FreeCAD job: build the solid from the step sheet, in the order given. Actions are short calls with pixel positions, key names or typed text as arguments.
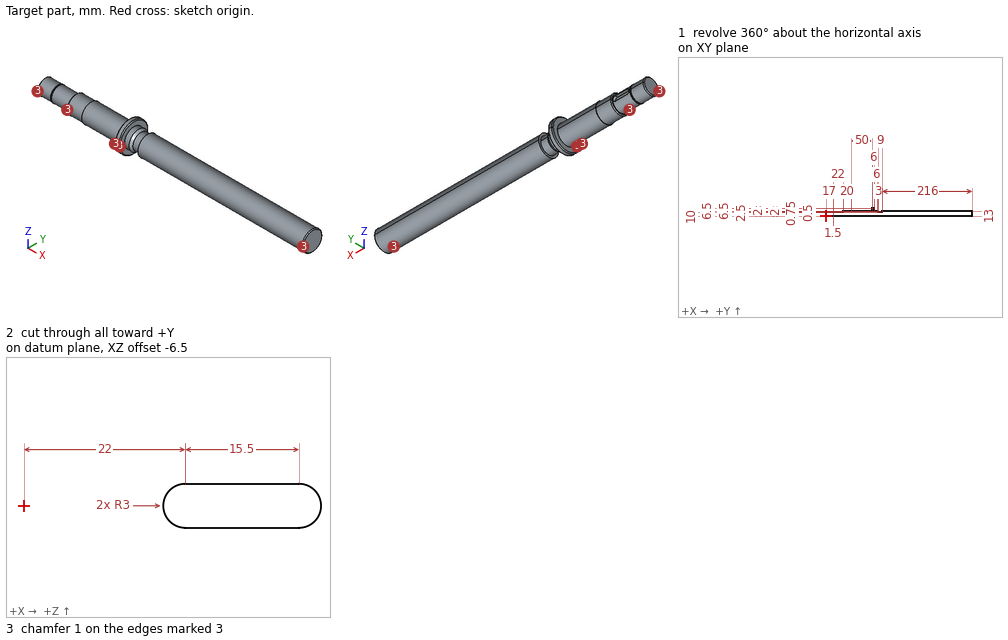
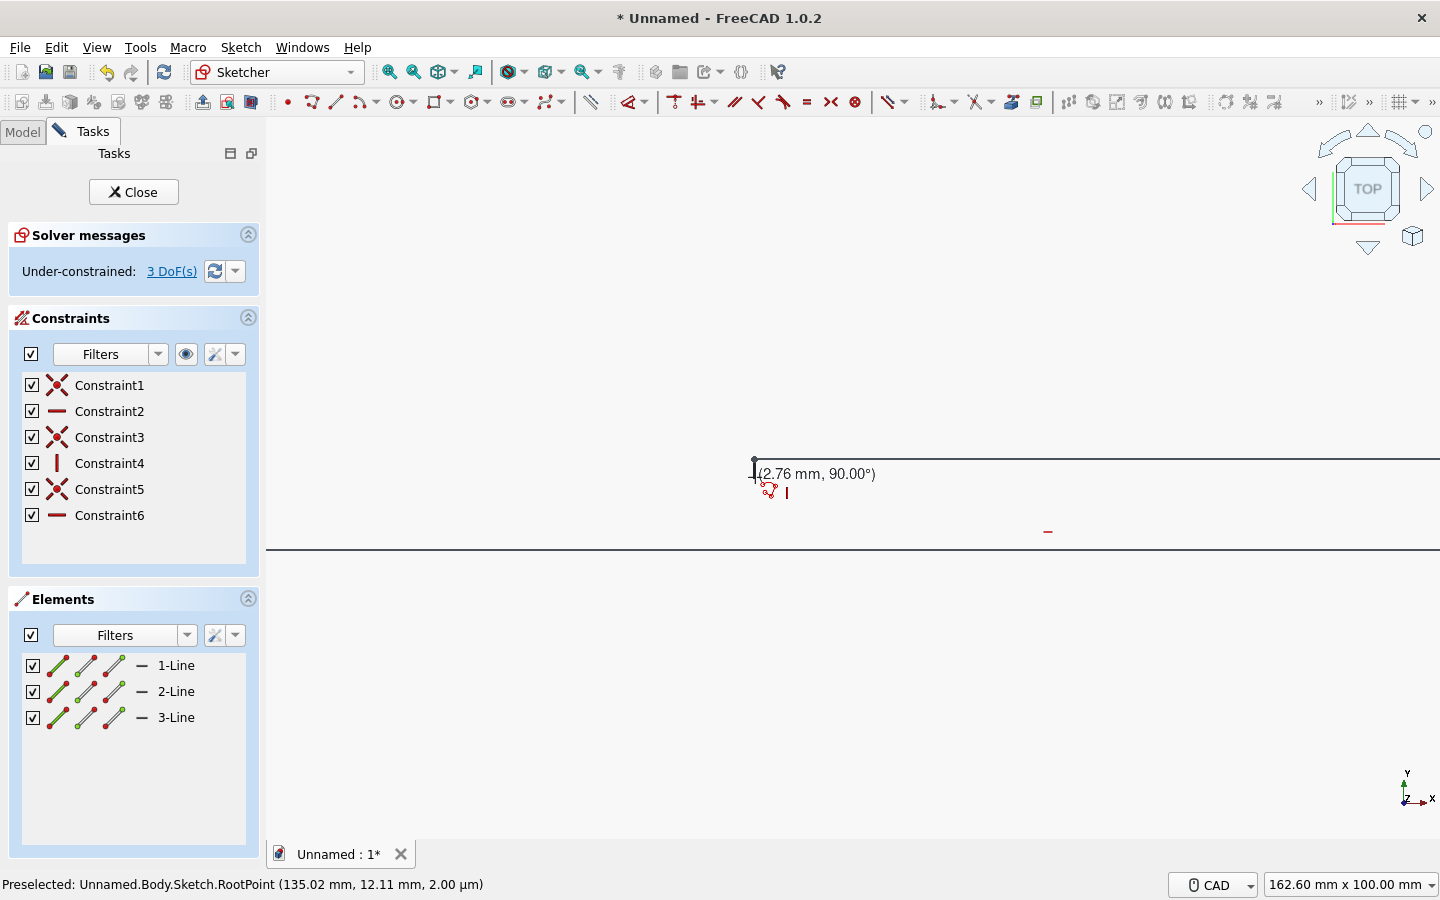
click(754, 474)
click(689, 474)
click(667, 460)
click(624, 460)
click(624, 413)
click(580, 413)
click(580, 460)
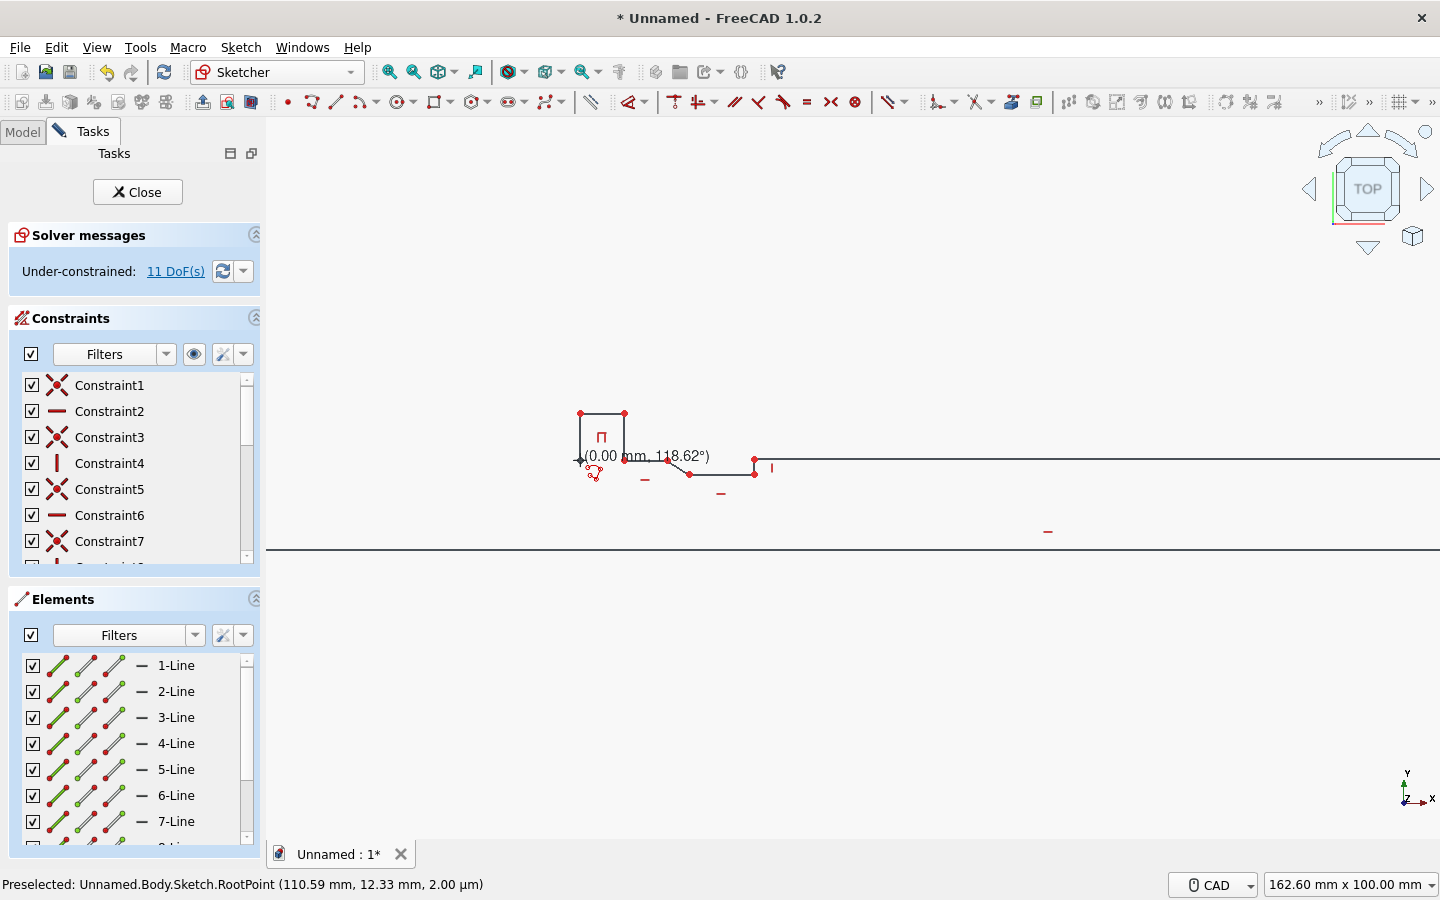
scroll(671, 477, down, 6)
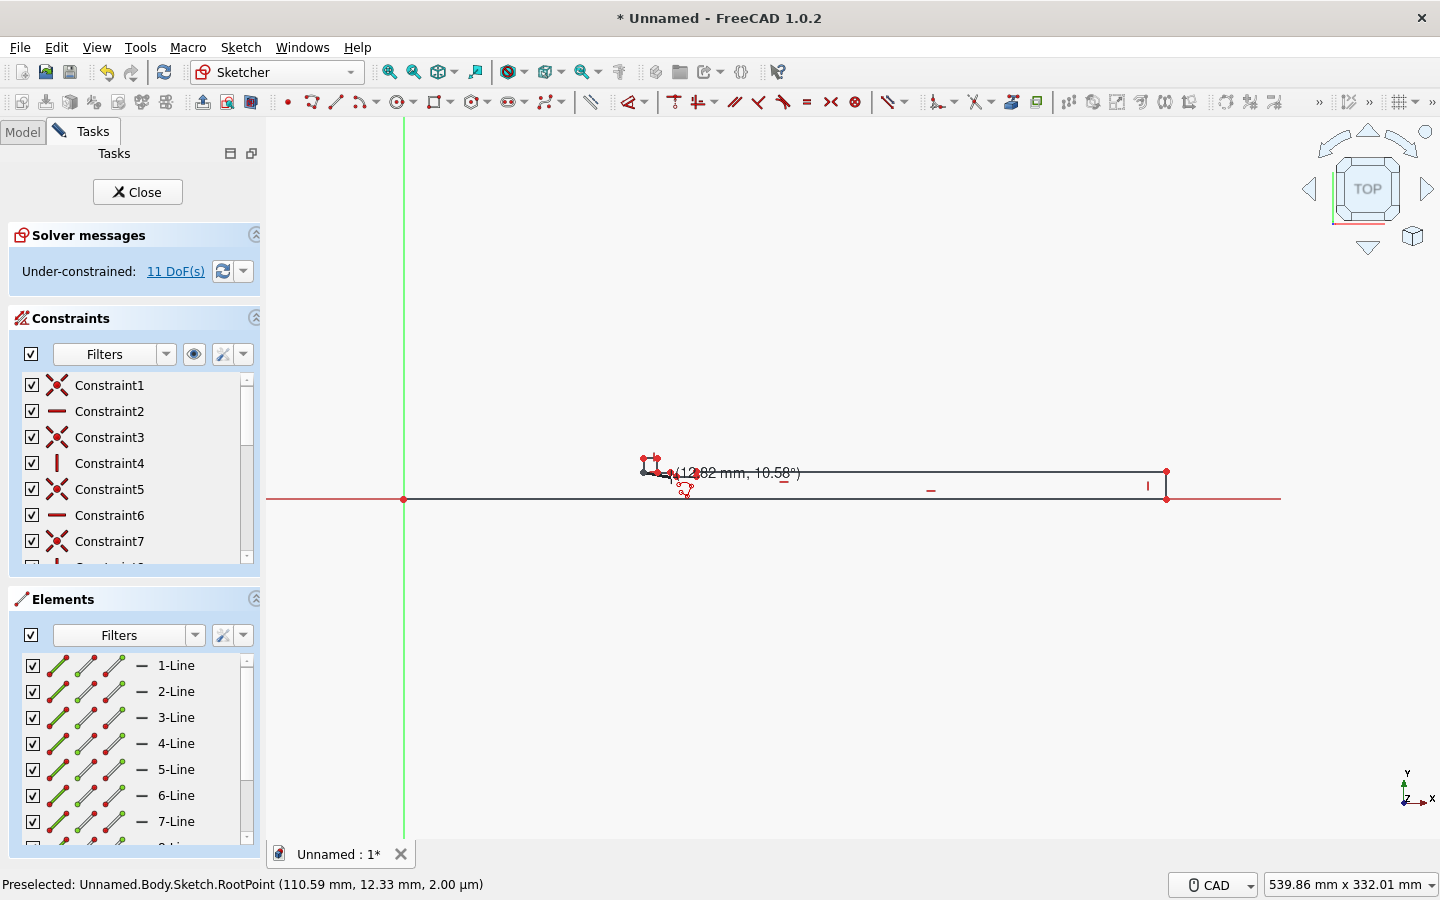
click(535, 472)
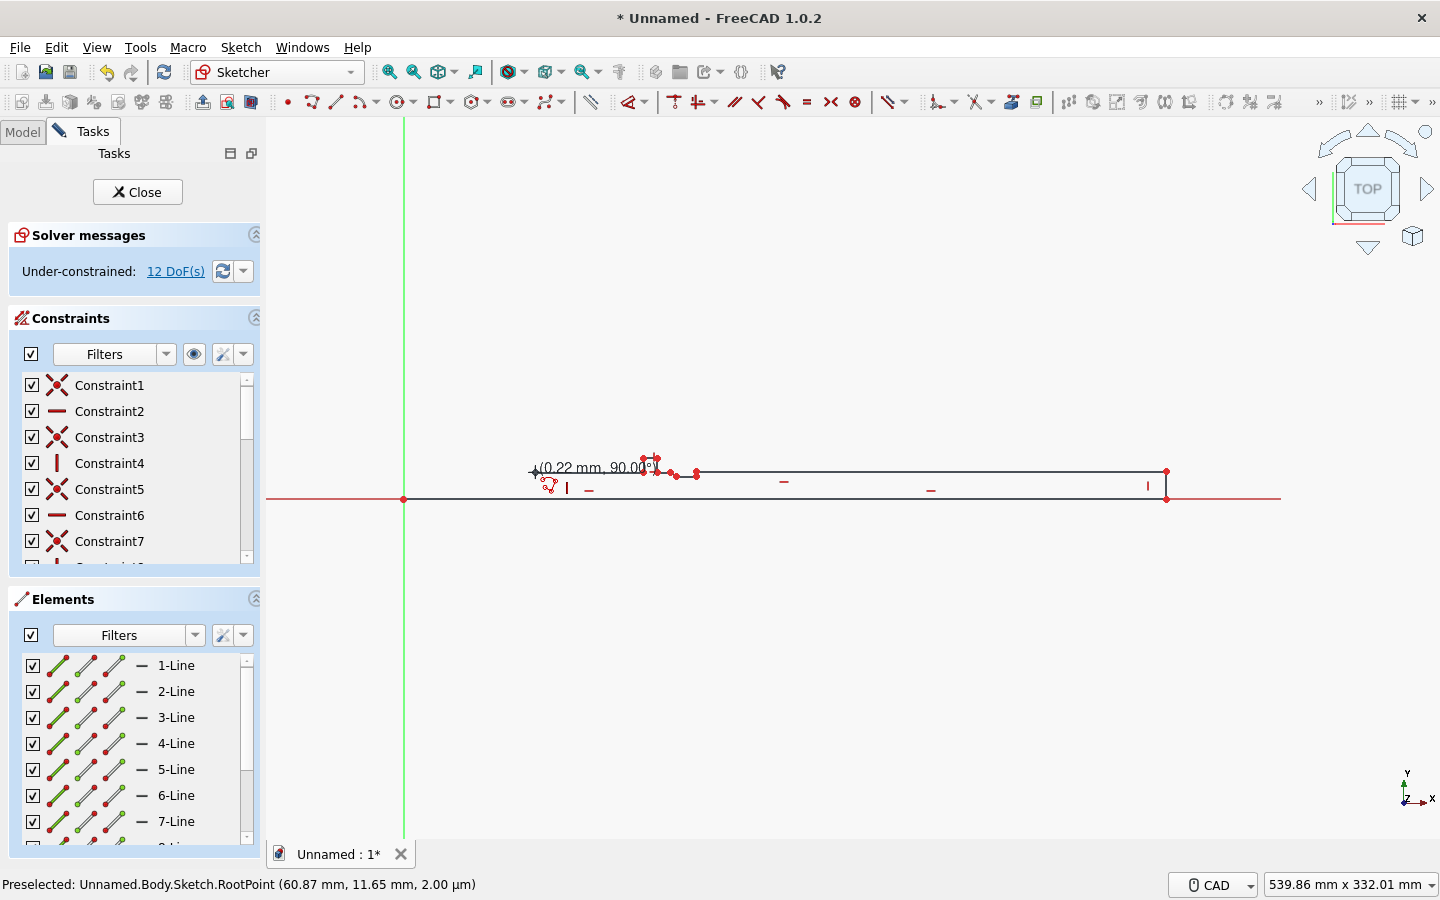
scroll(535, 473, up, 14)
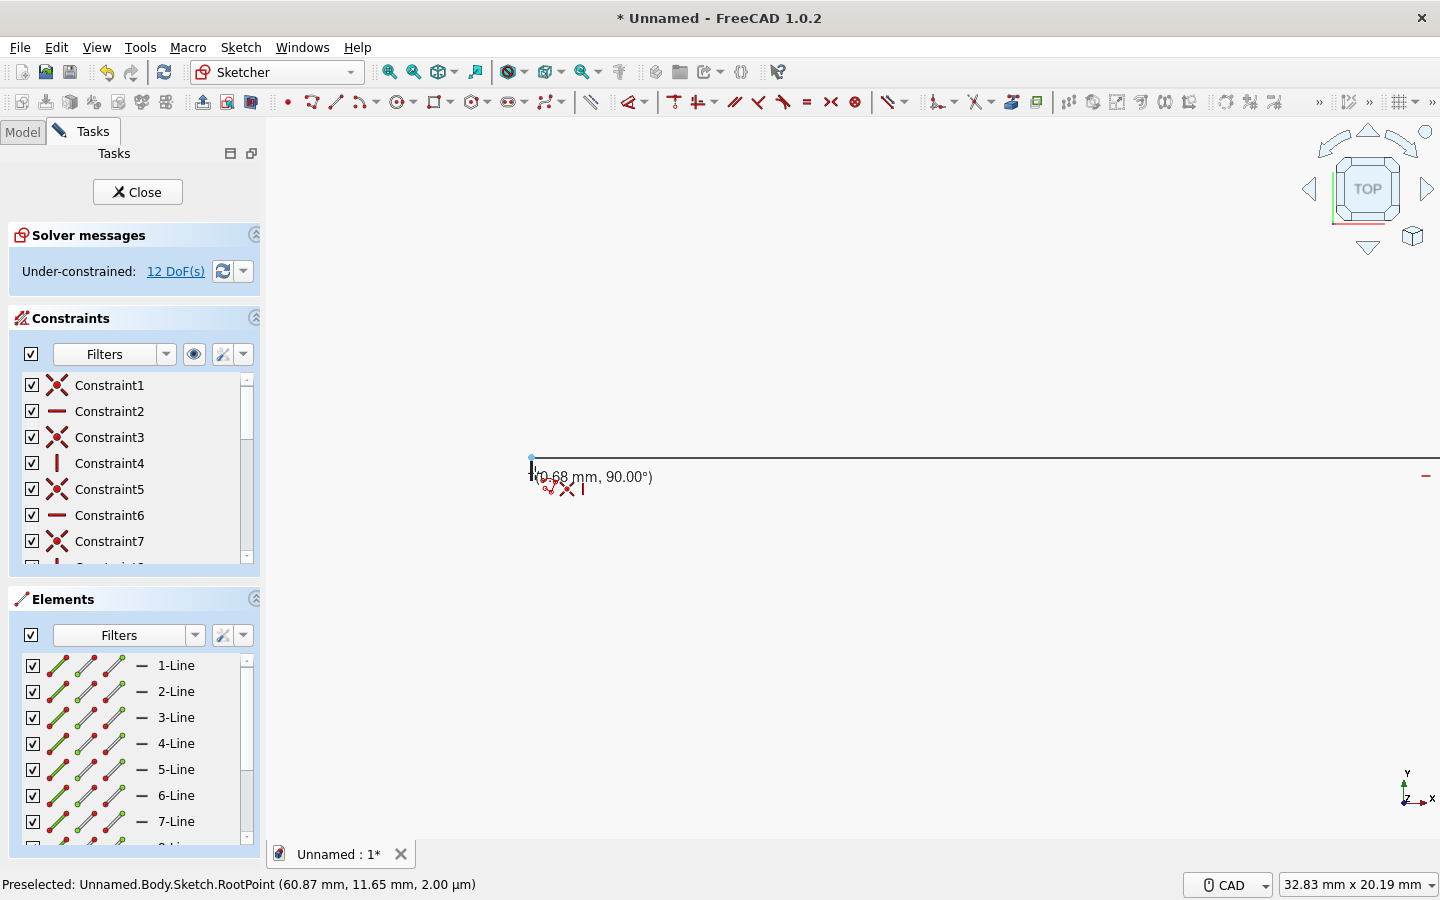
click(531, 469)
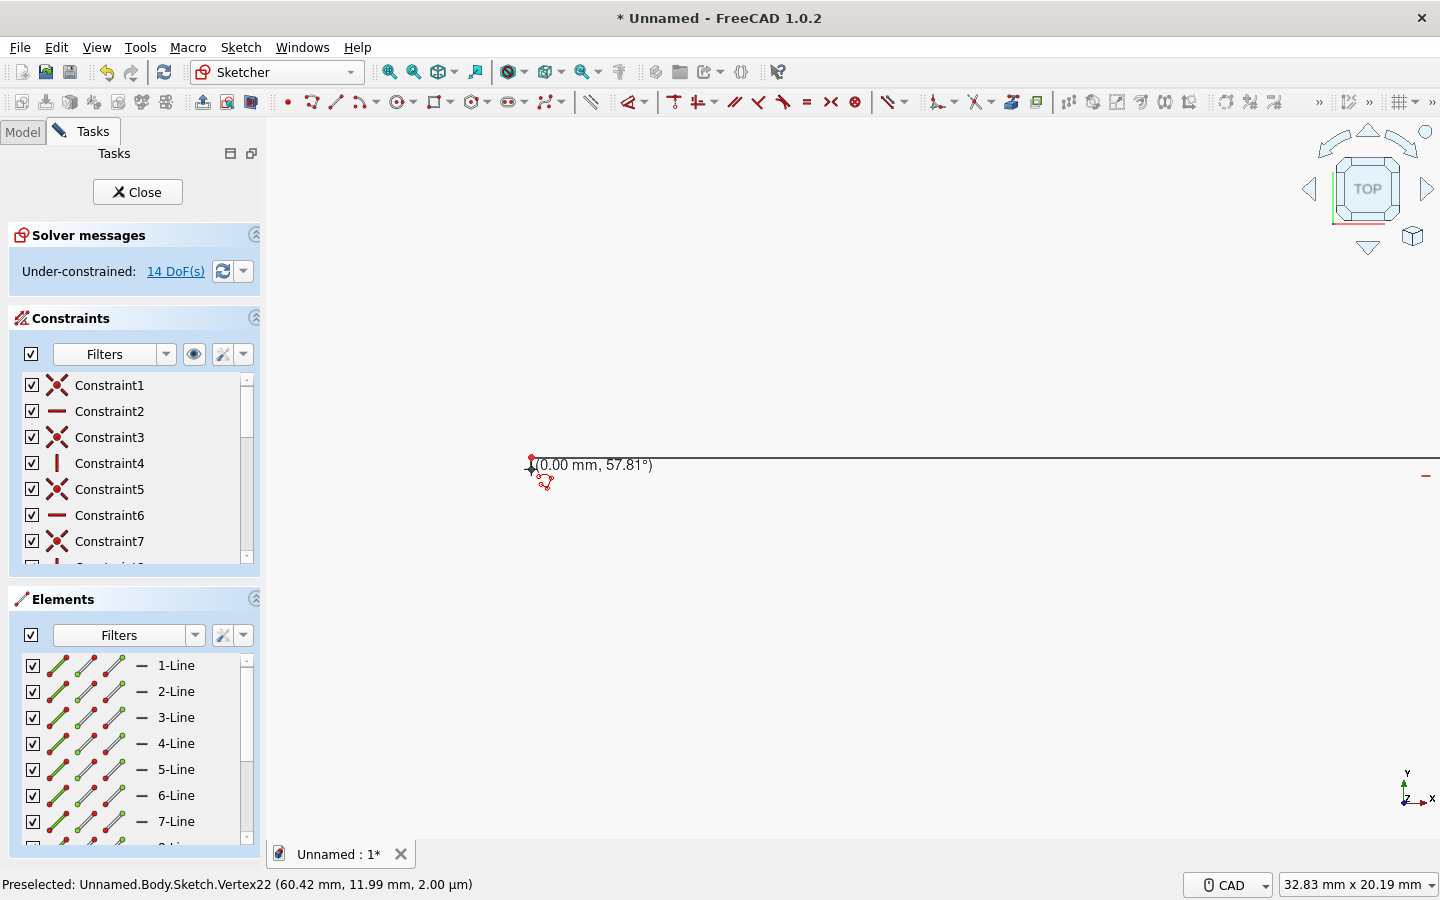
scroll(535, 473, down, 14)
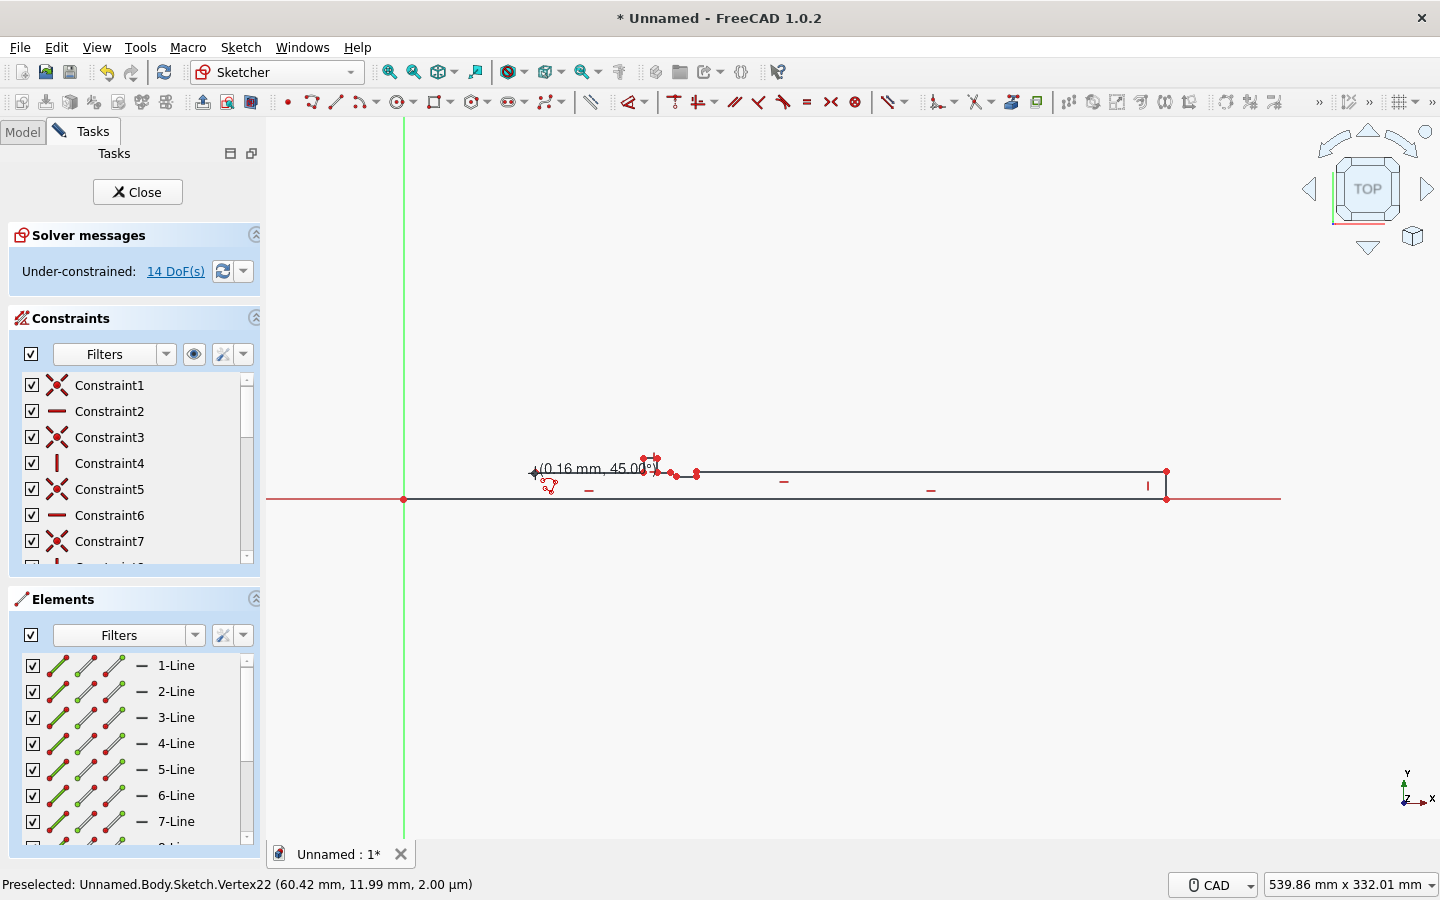
click(492, 473)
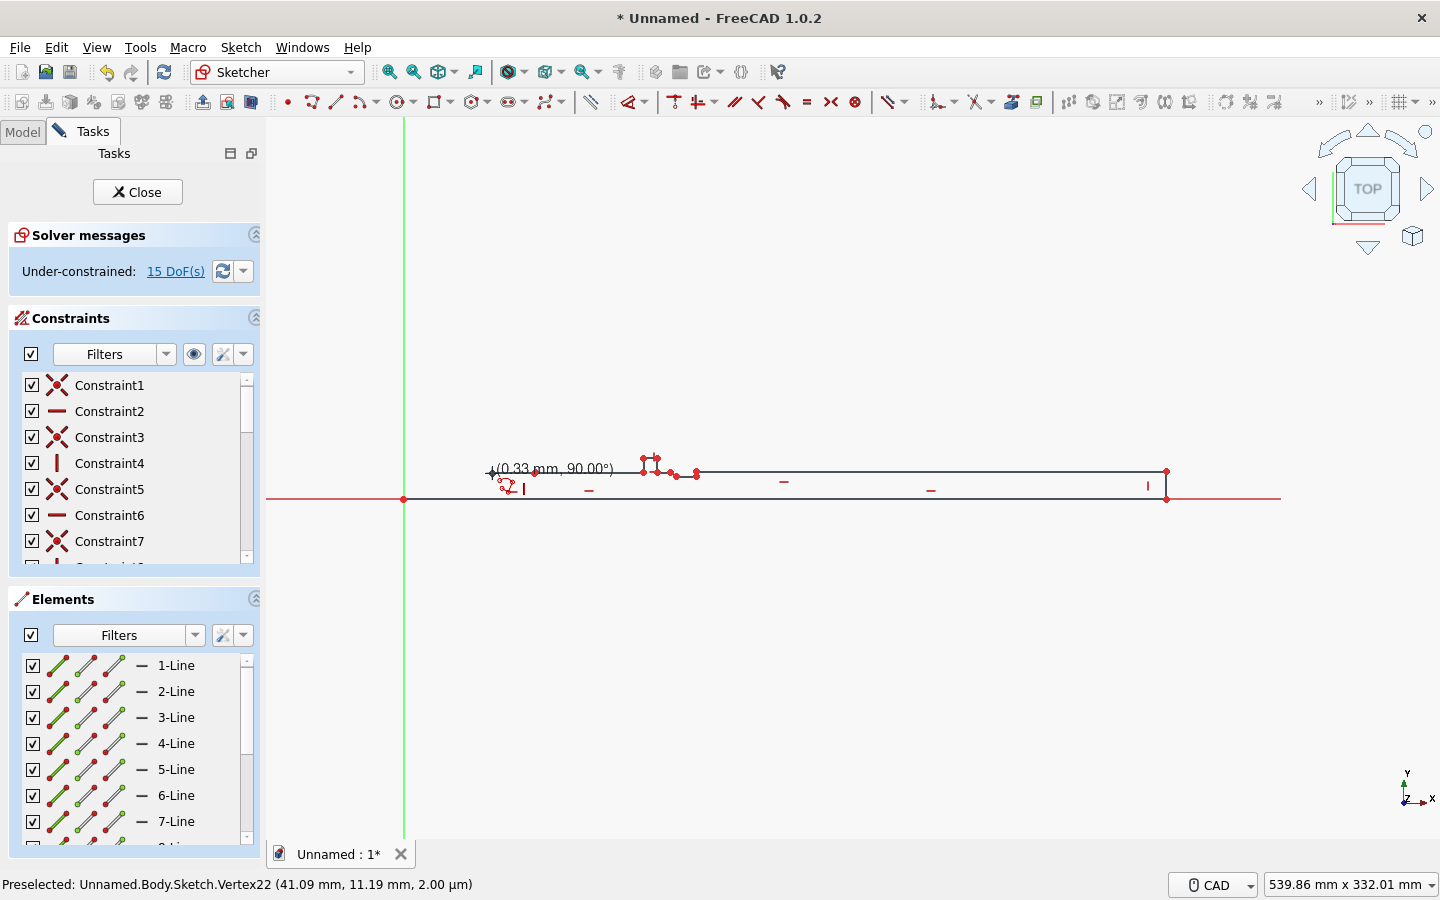
scroll(492, 478, up, 7)